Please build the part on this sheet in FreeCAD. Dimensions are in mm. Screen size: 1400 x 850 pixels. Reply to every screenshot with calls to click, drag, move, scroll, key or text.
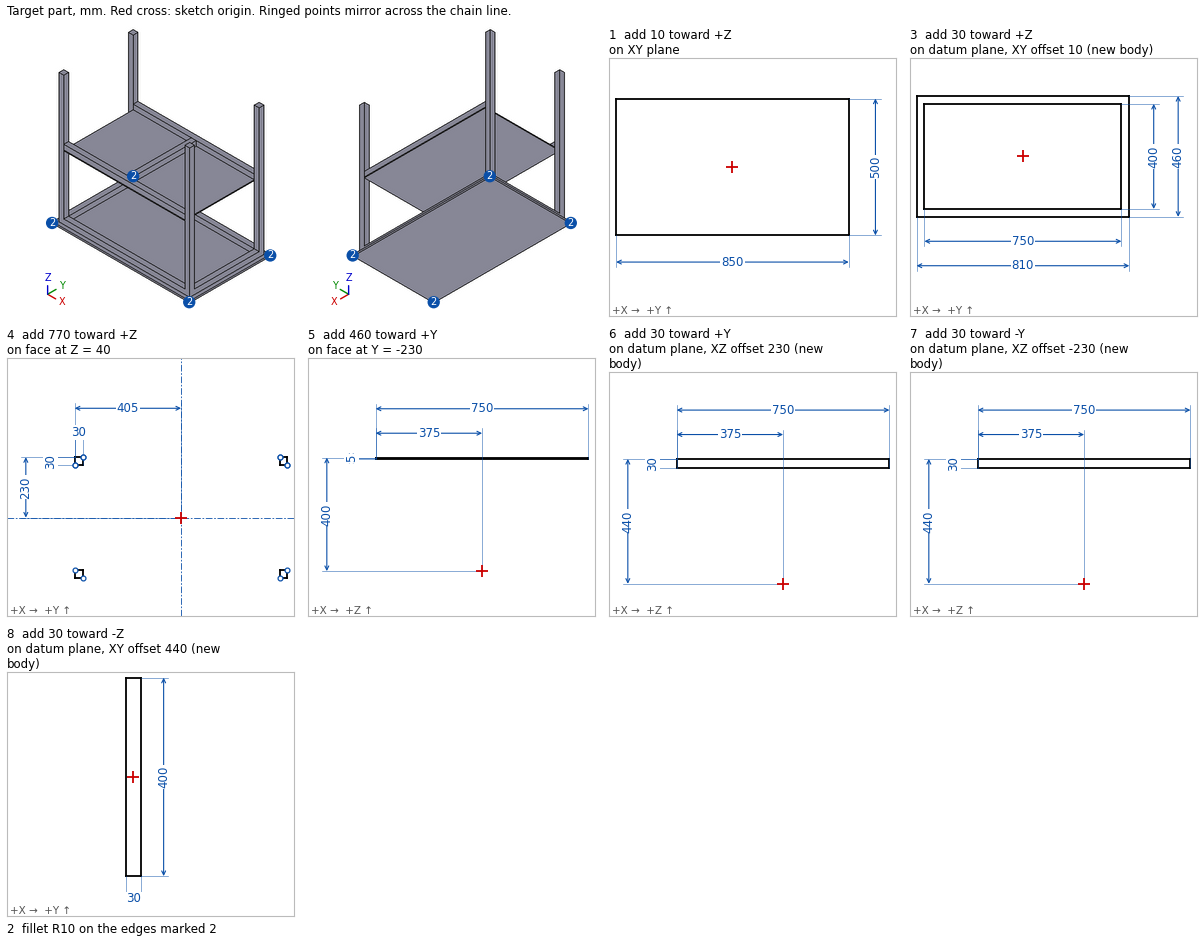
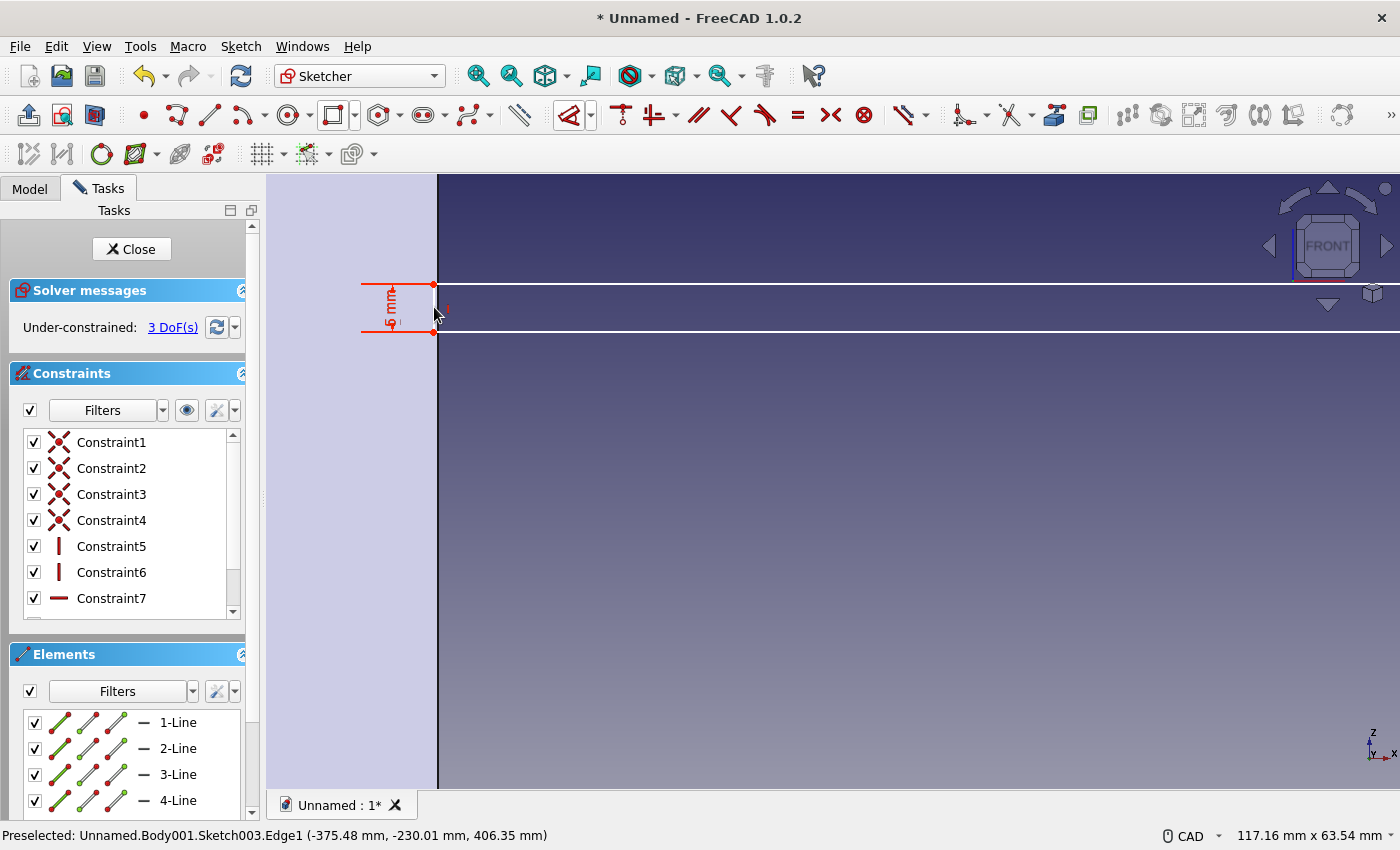
scroll(435, 309, down, 12)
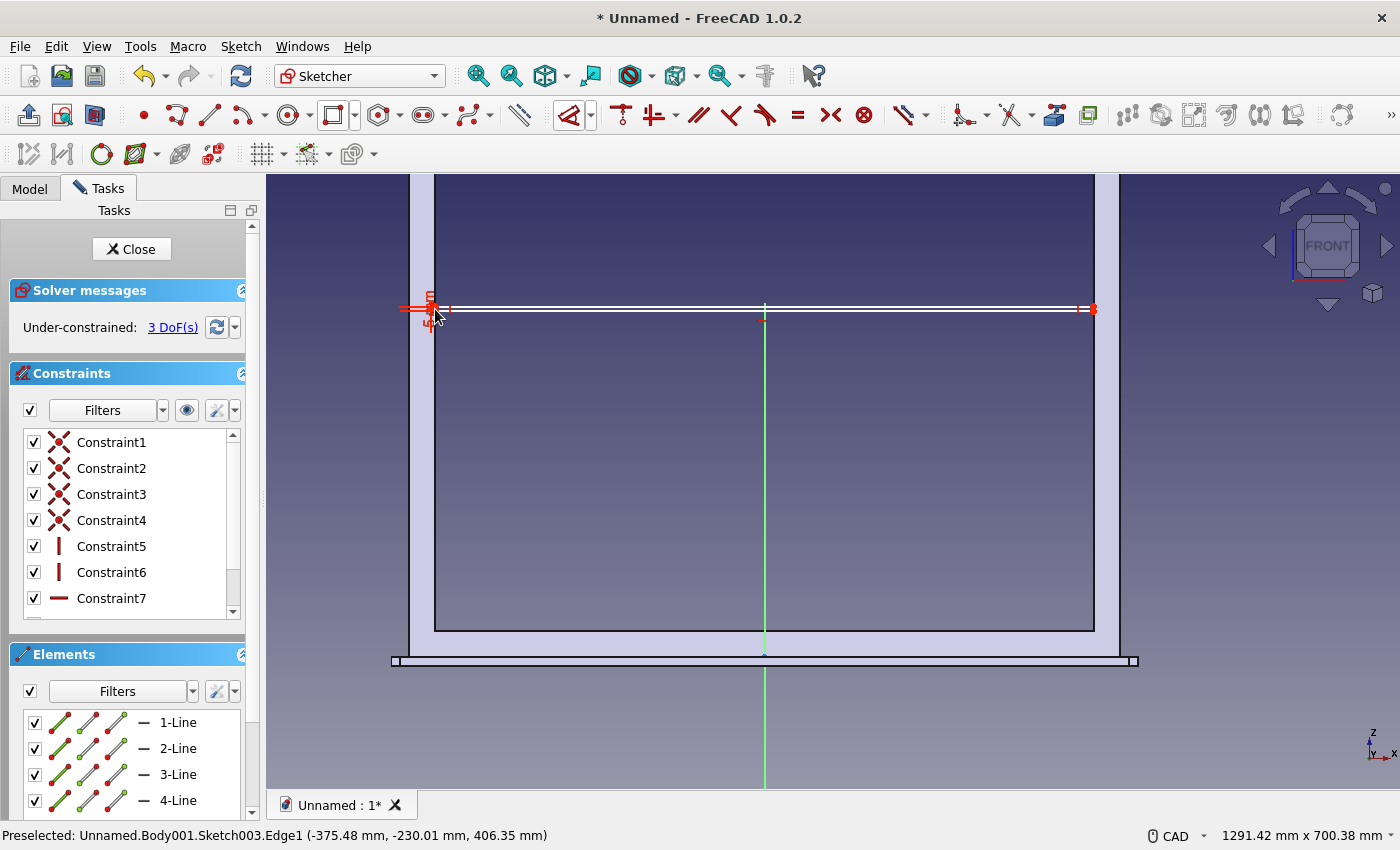
scroll(633, 311, up, 6)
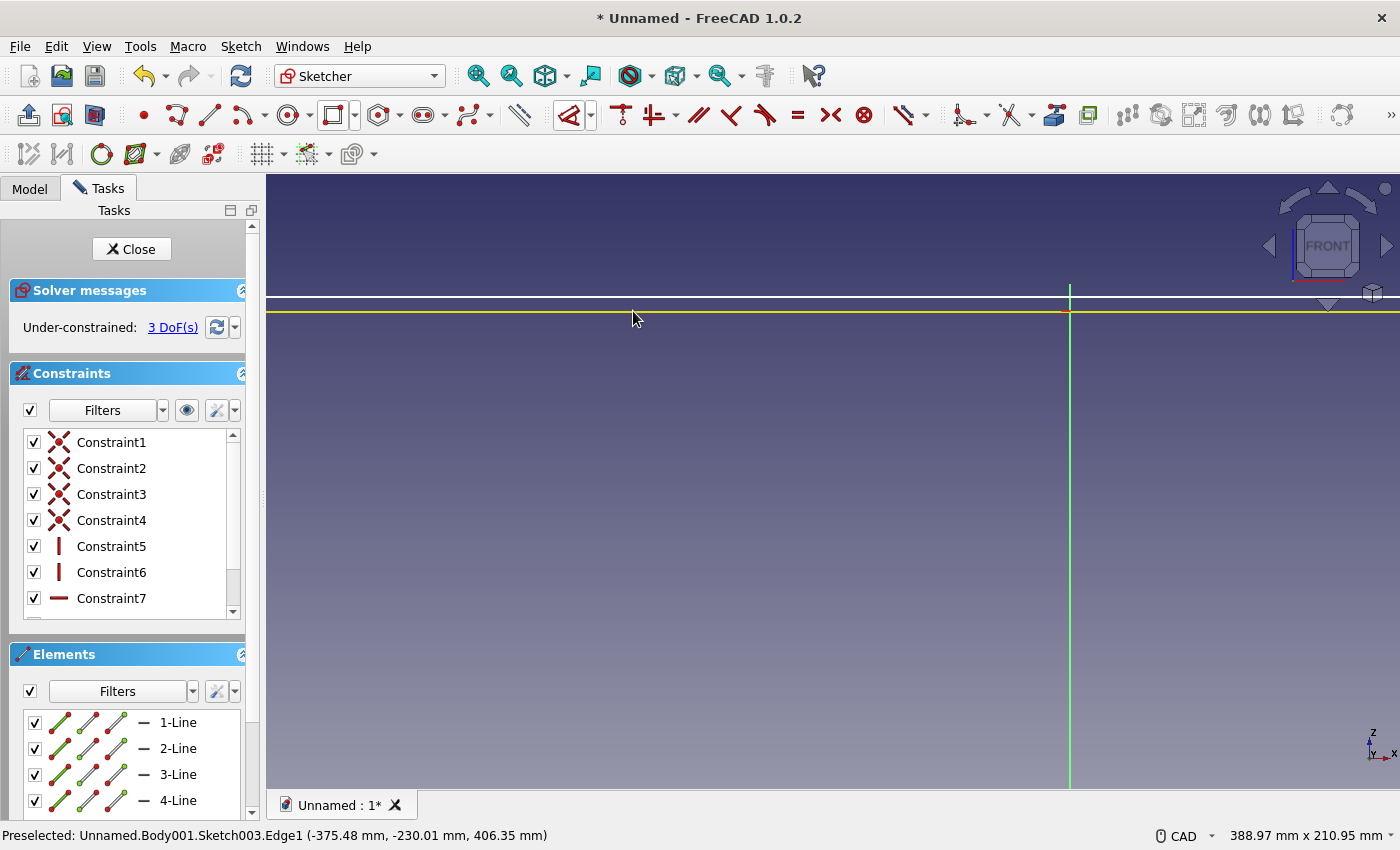
click(631, 312)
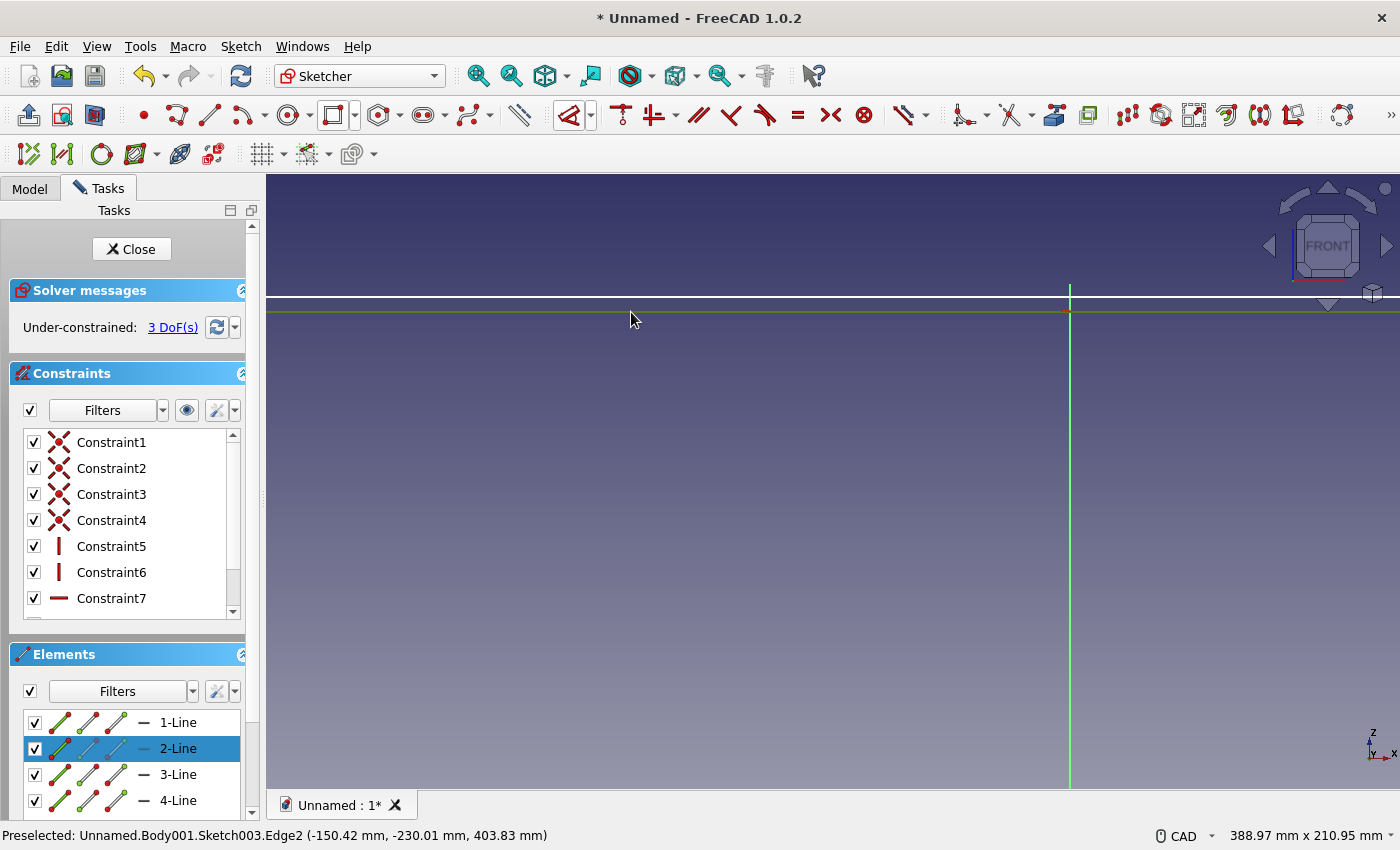
key(l)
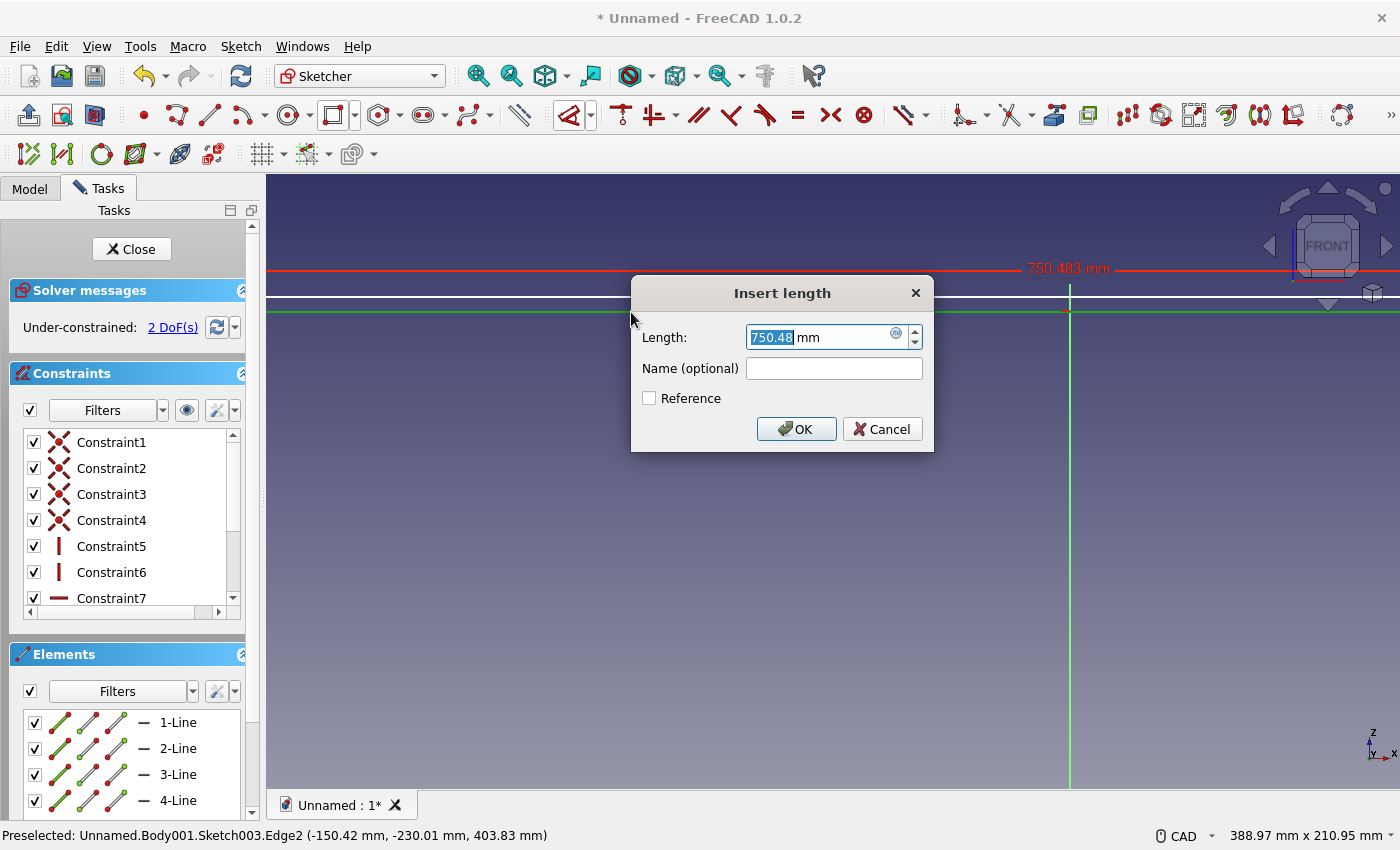
text(750)
key(Return)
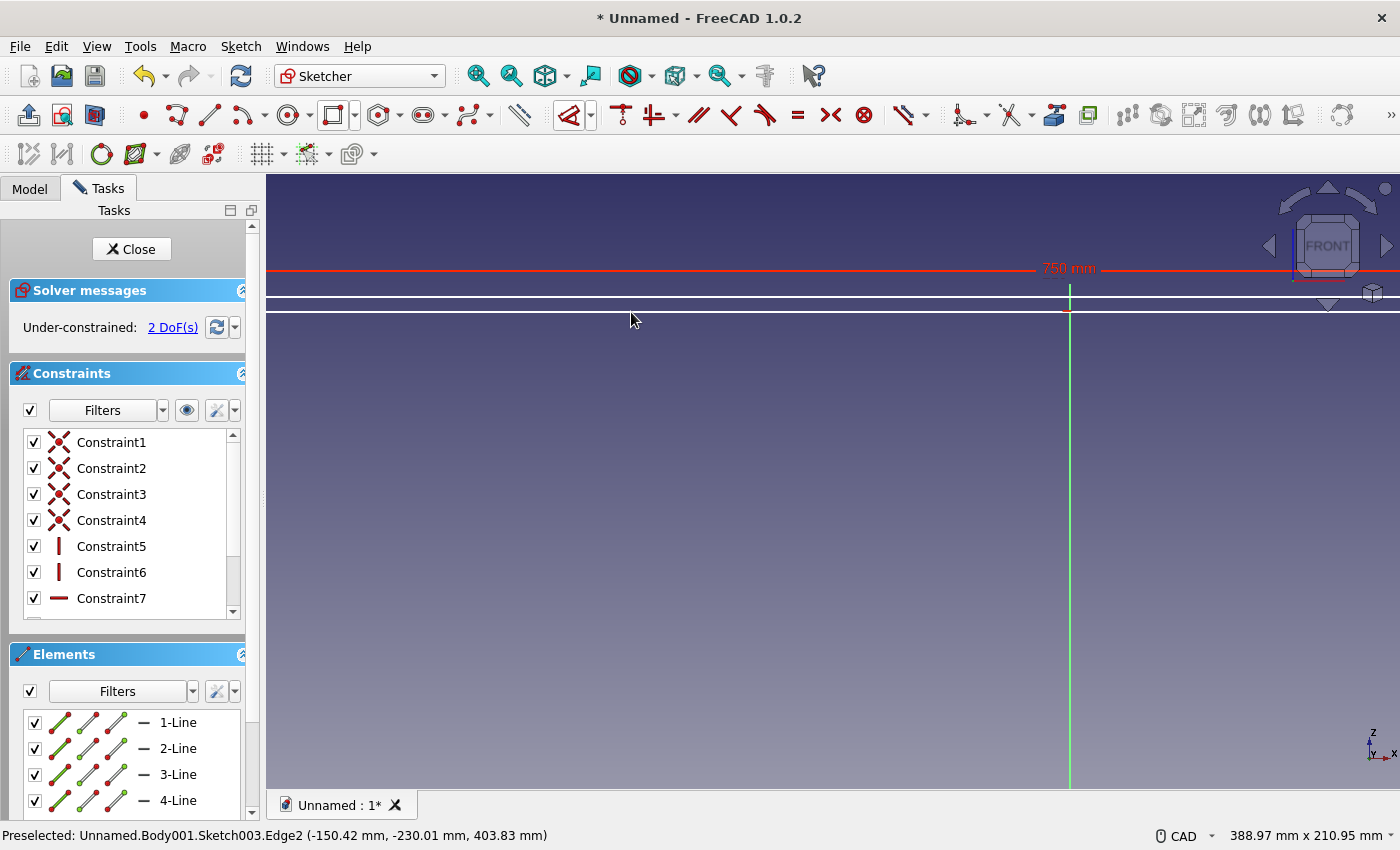
scroll(633, 311, down, 6)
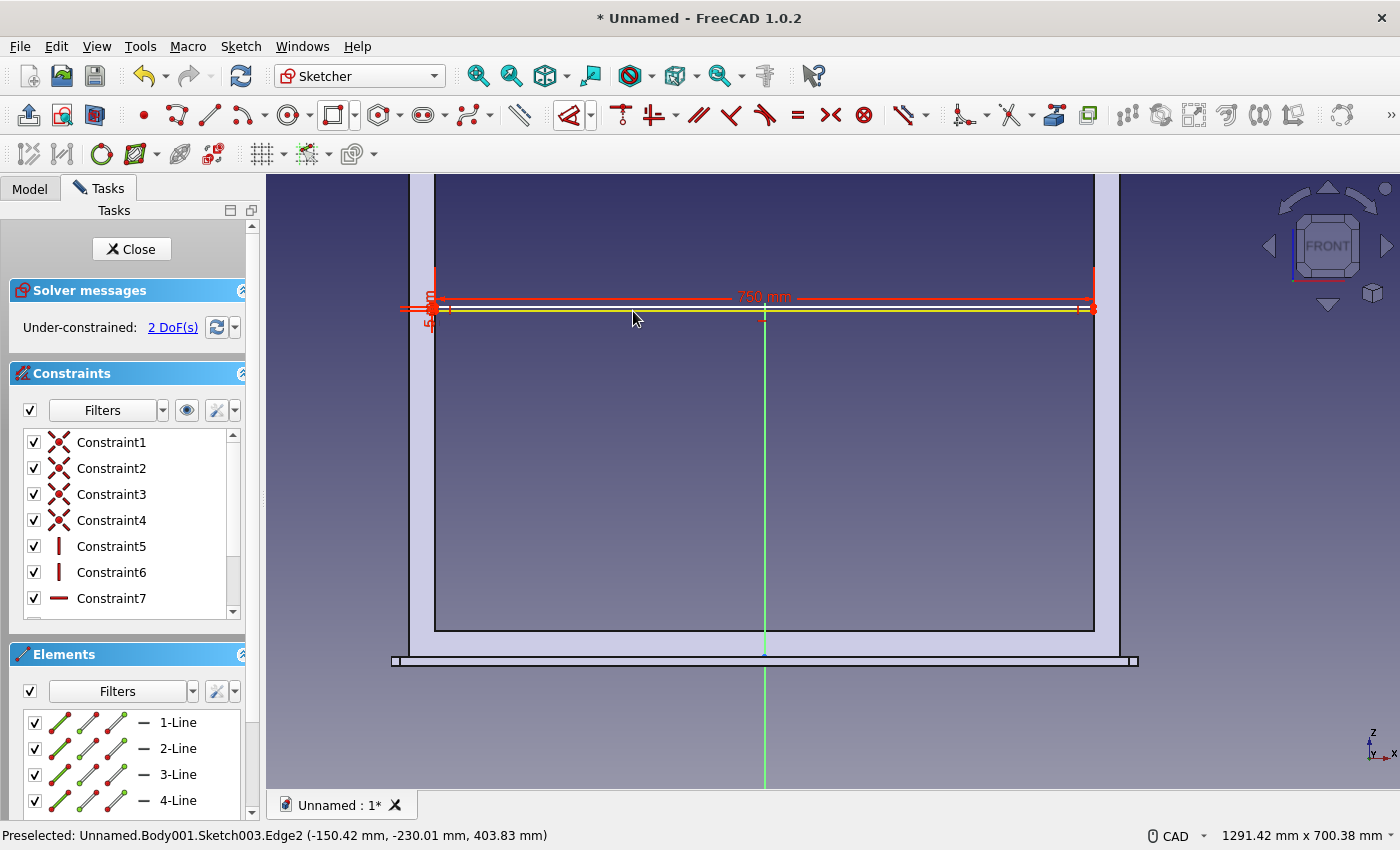
scroll(435, 307, up, 6)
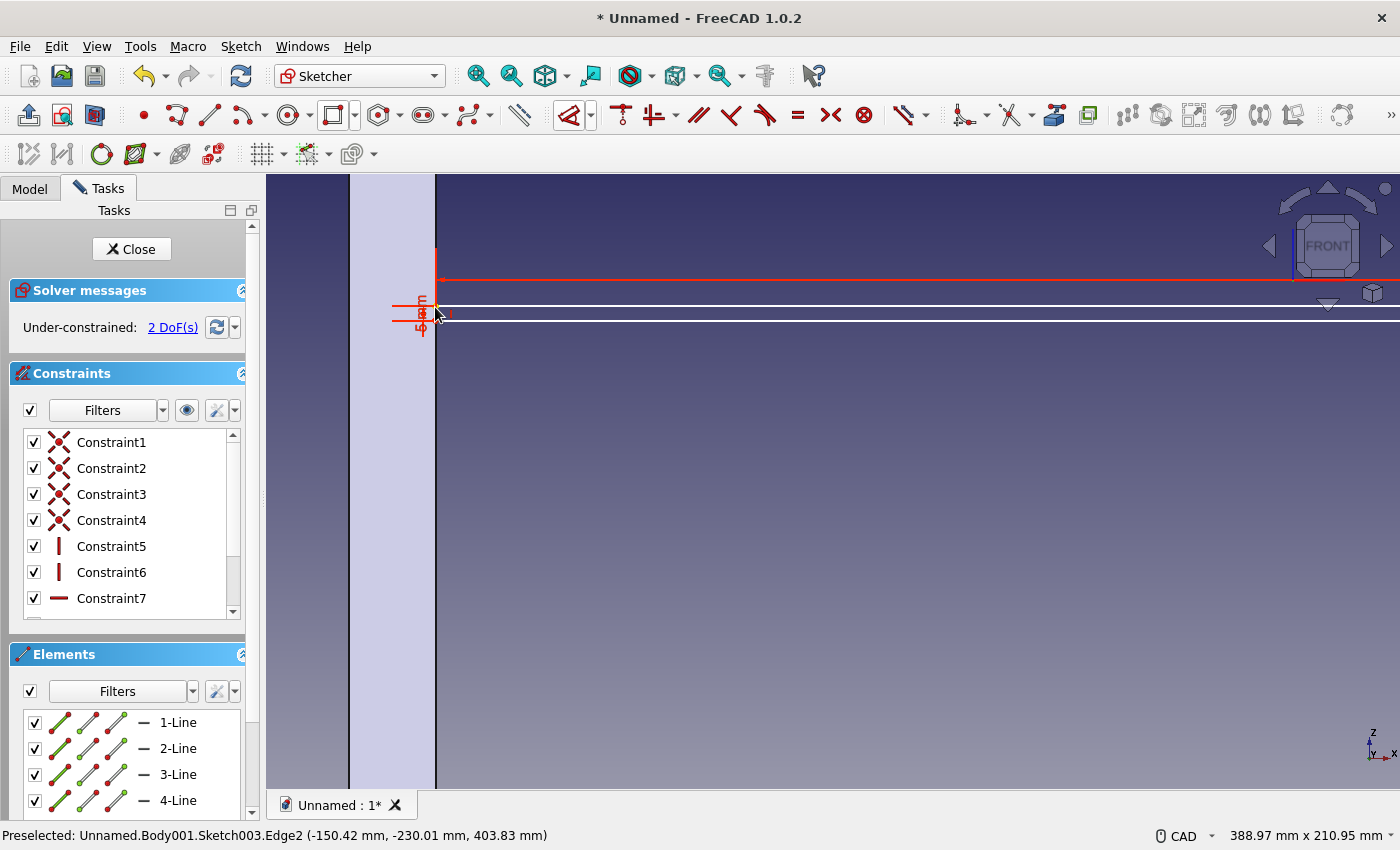
click(436, 306)